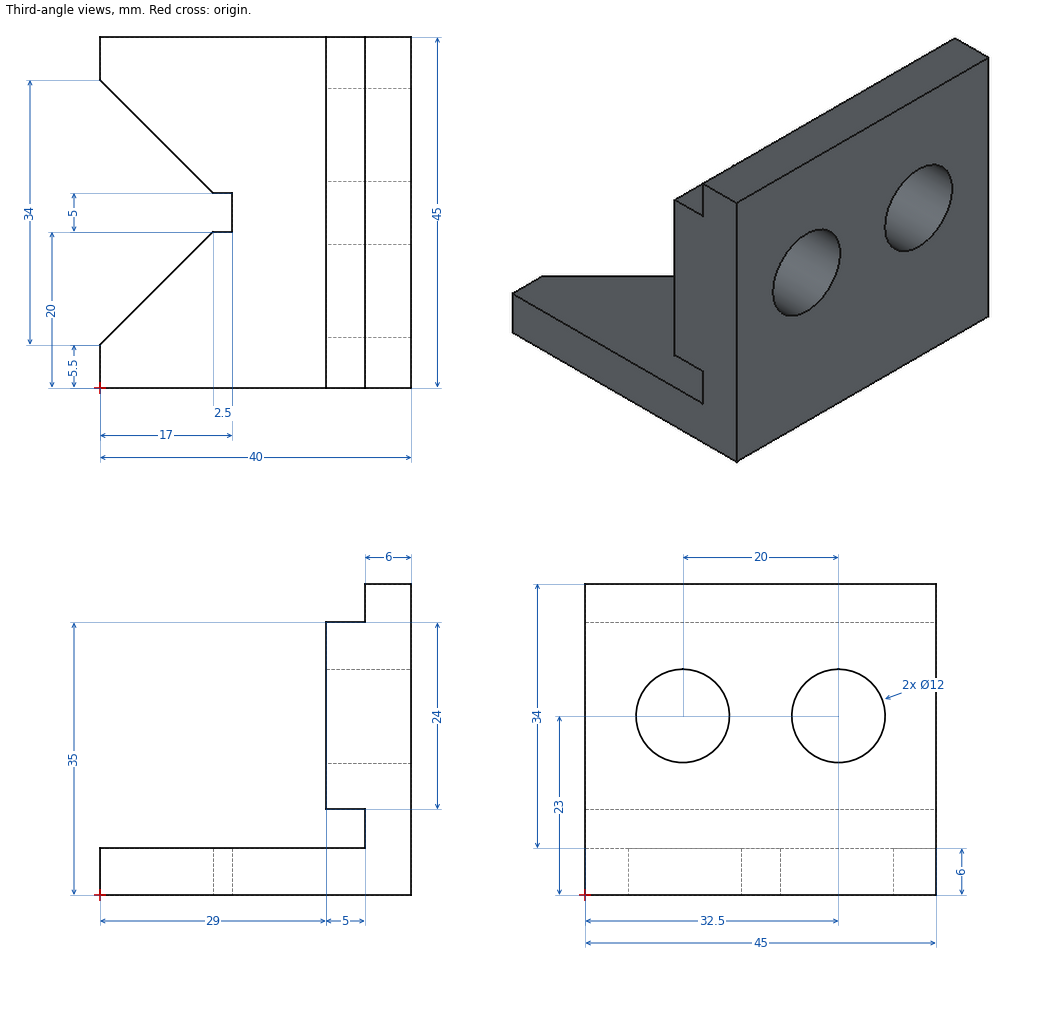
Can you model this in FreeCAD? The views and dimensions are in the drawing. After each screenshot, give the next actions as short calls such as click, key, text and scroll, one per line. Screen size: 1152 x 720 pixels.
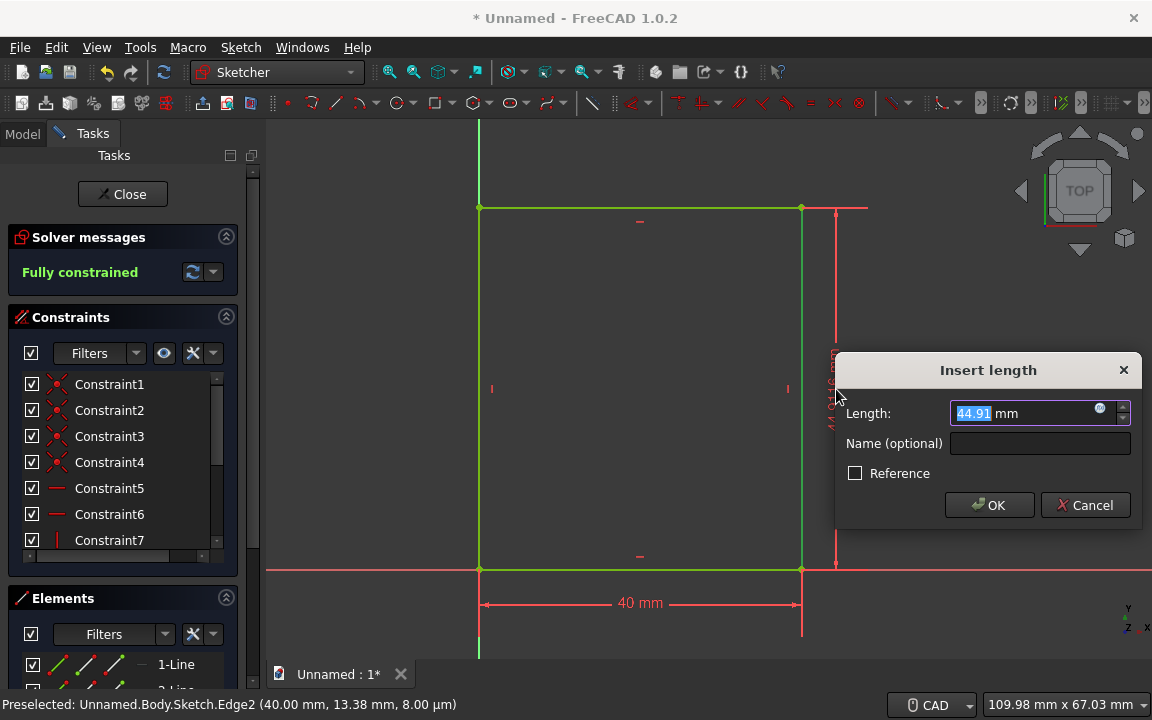
text(45)
key(Return)
key(Escape)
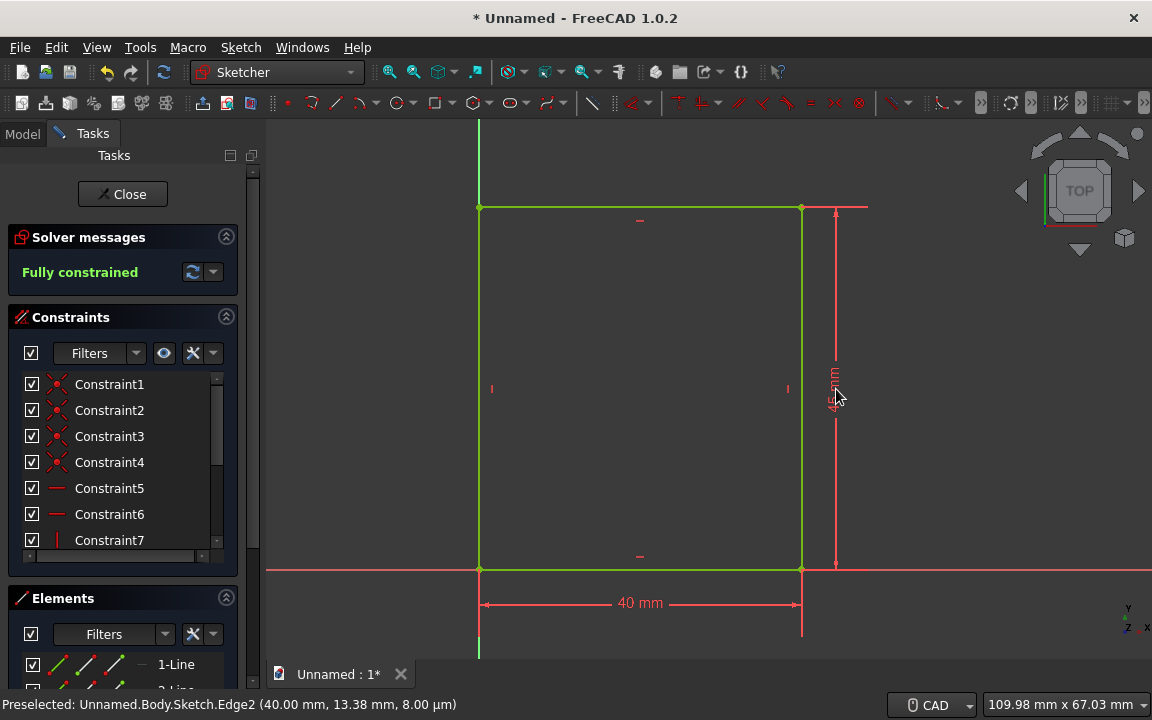
click(123, 194)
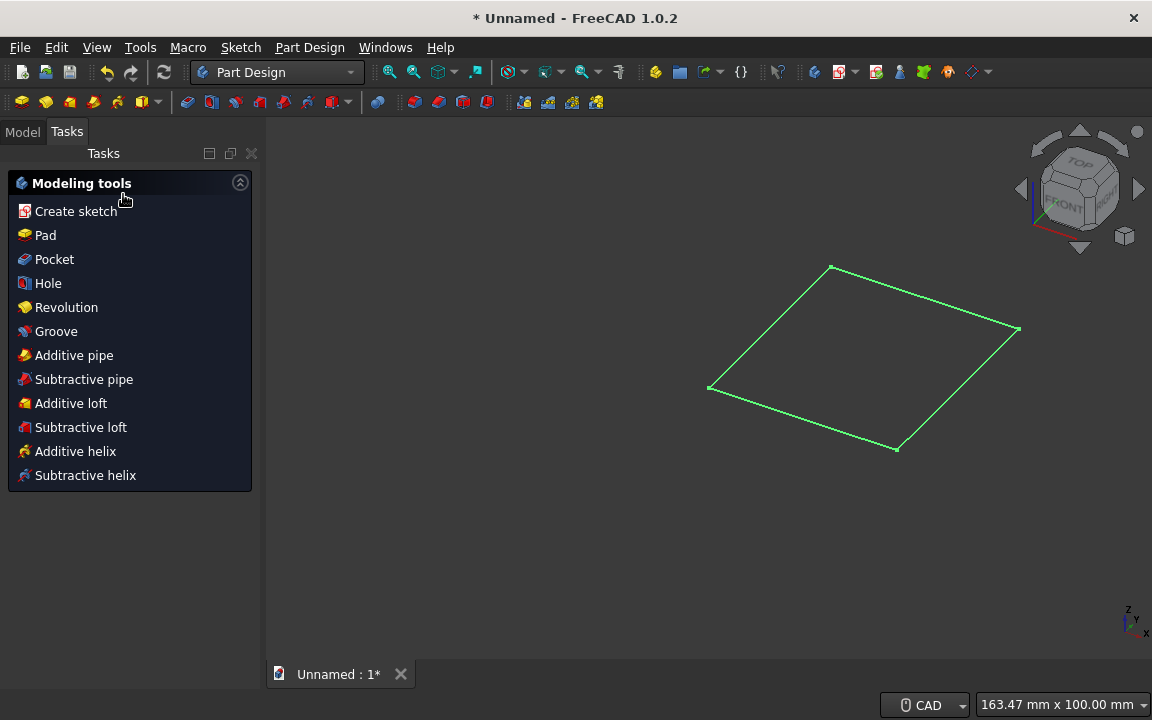
click(22, 102)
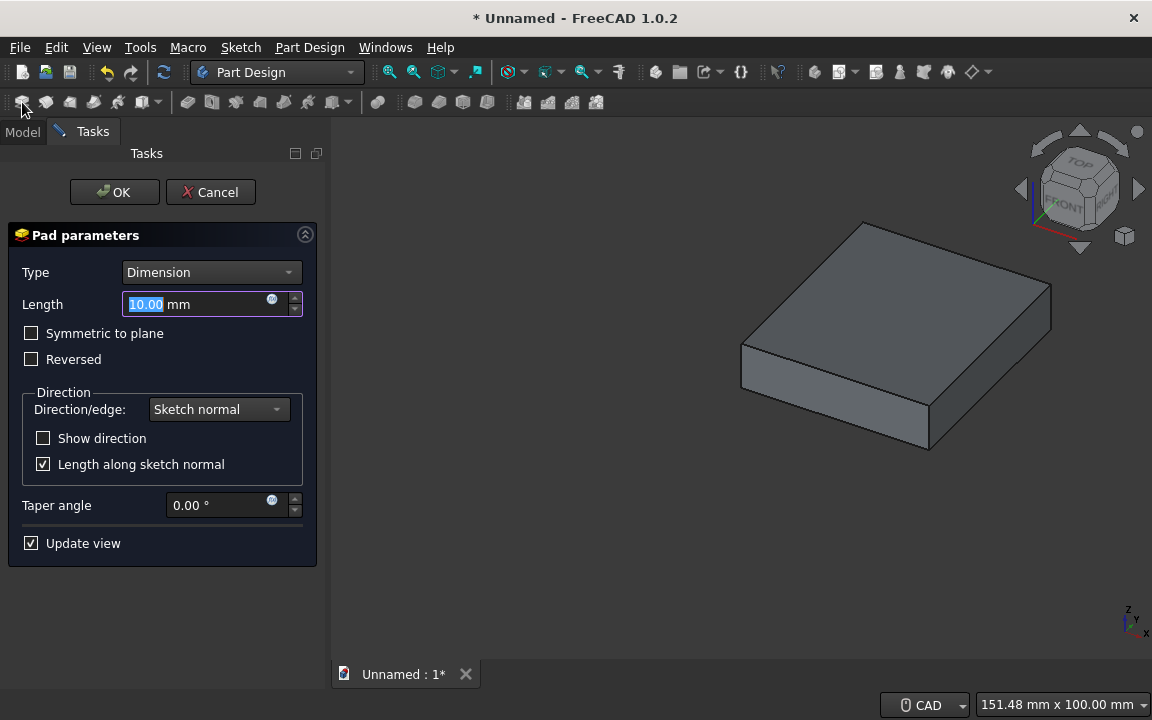
text(6)
key(Tab)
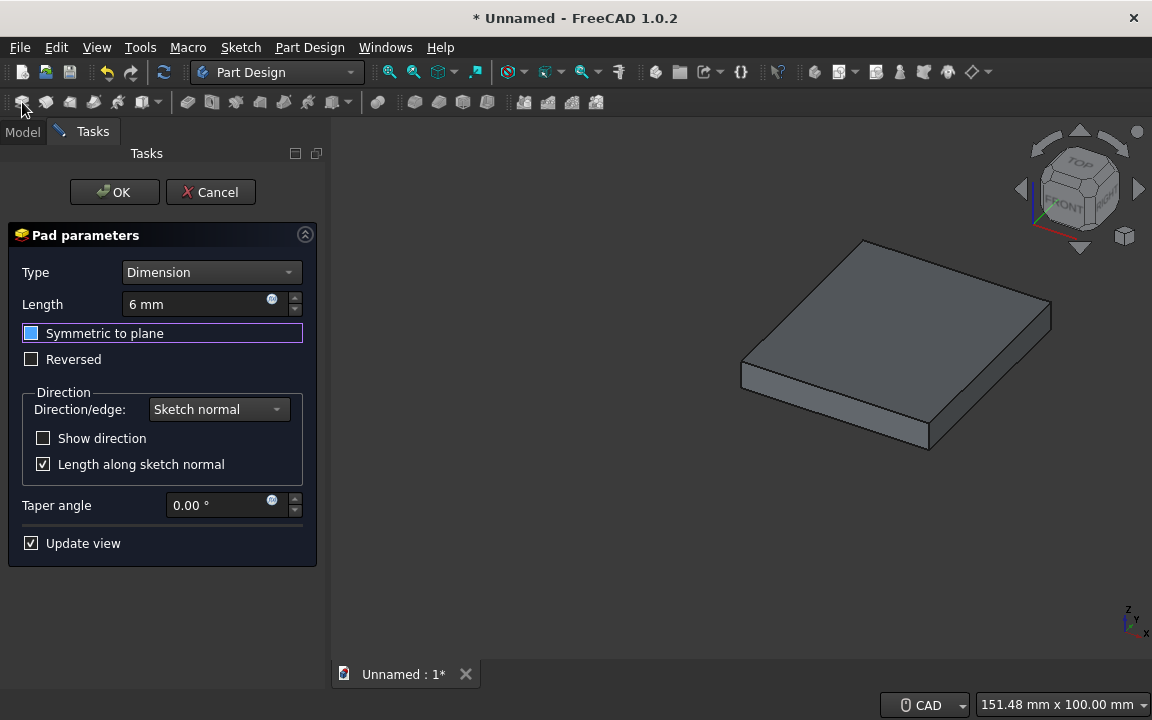
click(115, 192)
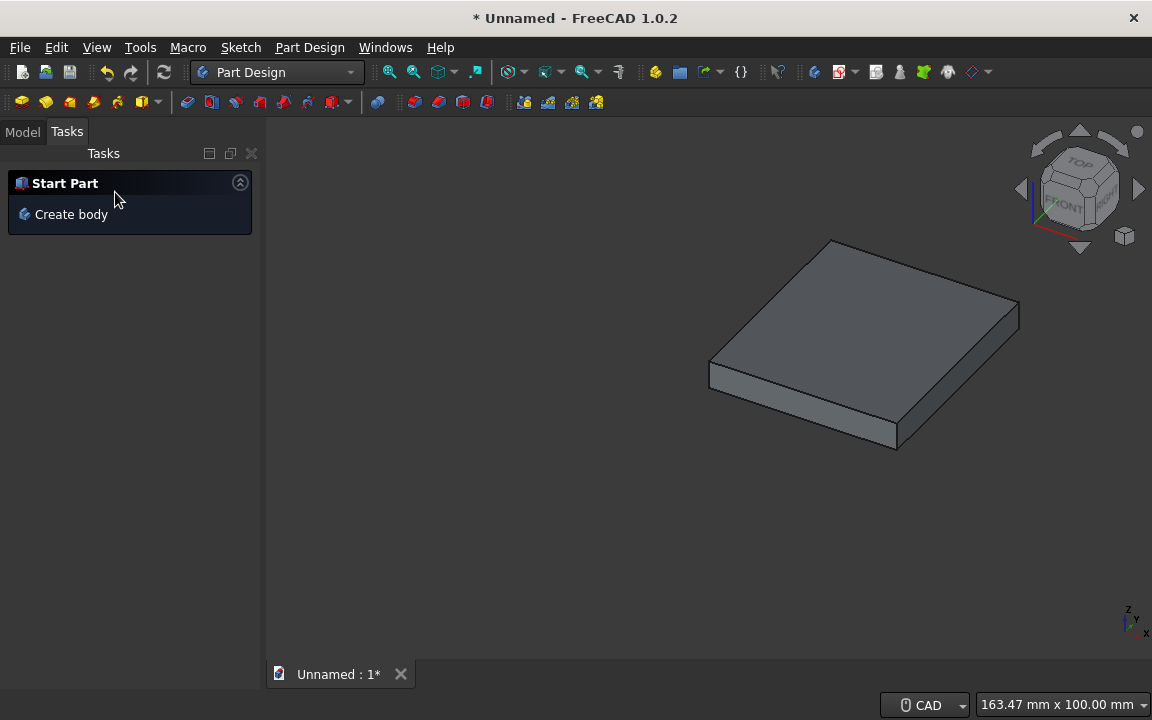
click(390, 72)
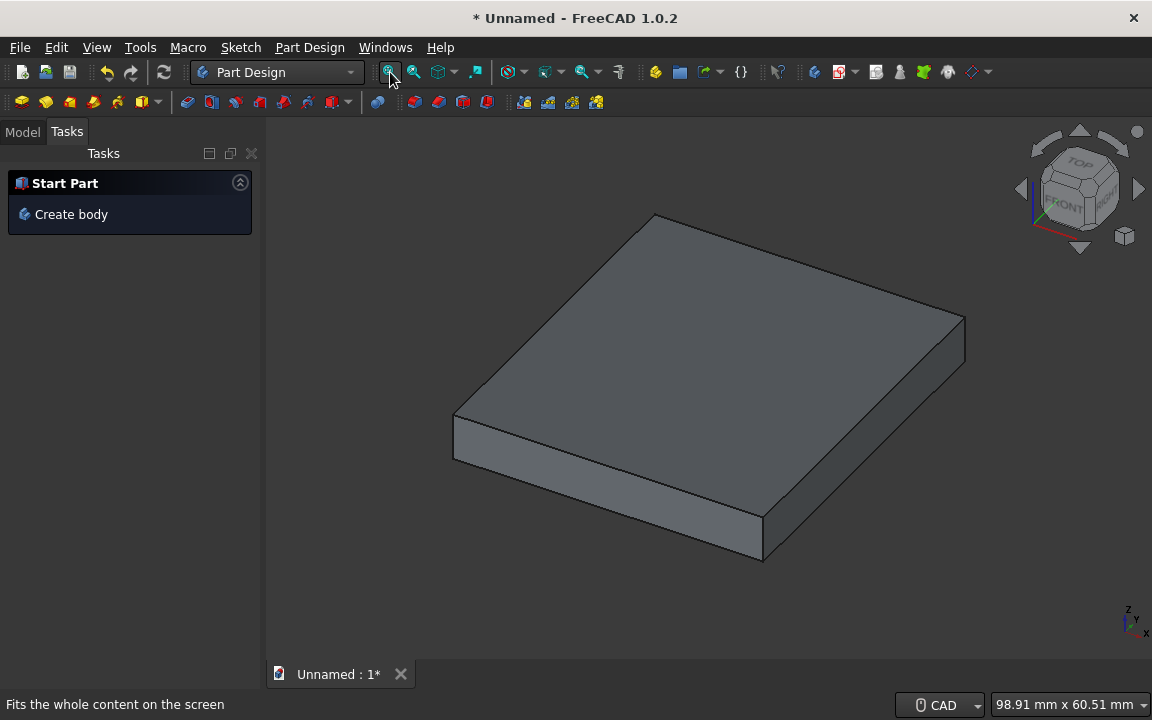
click(951, 353)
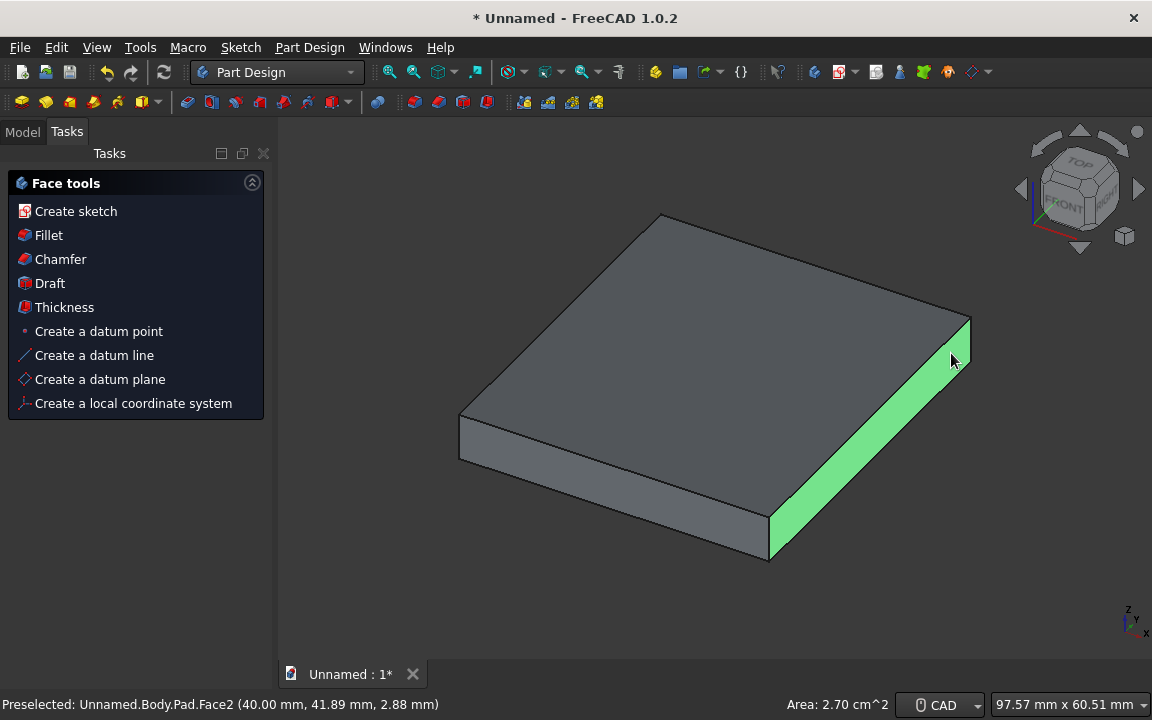
click(840, 72)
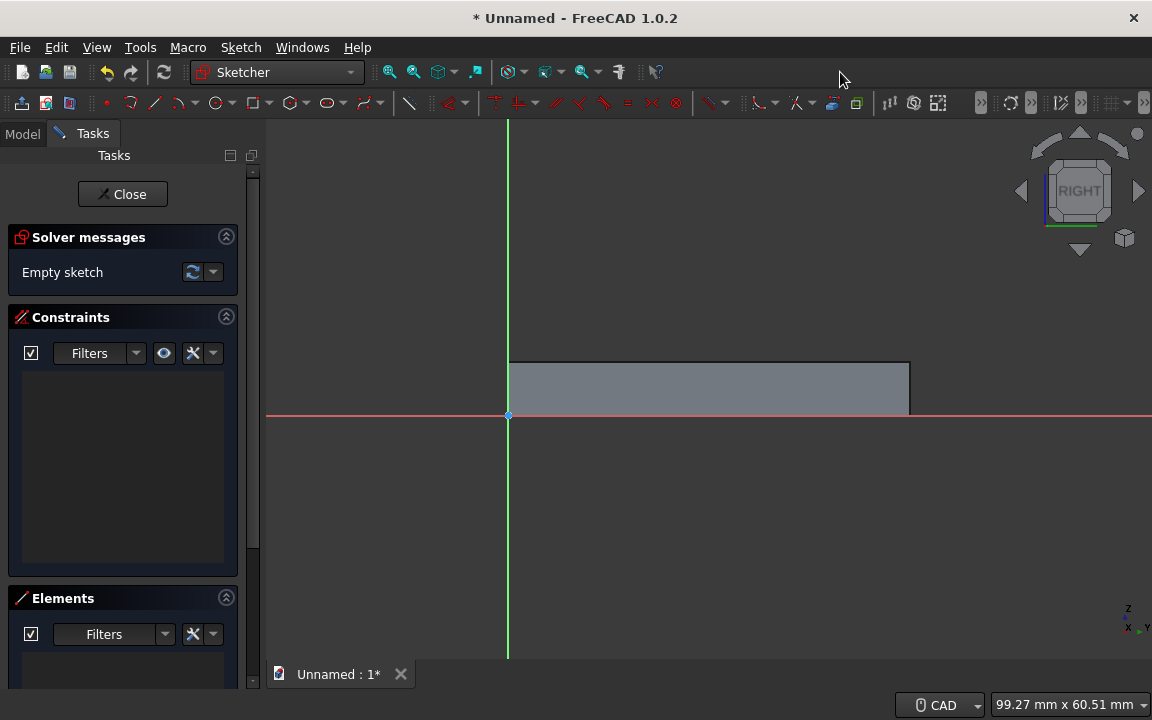
scroll(501, 631, down, 2)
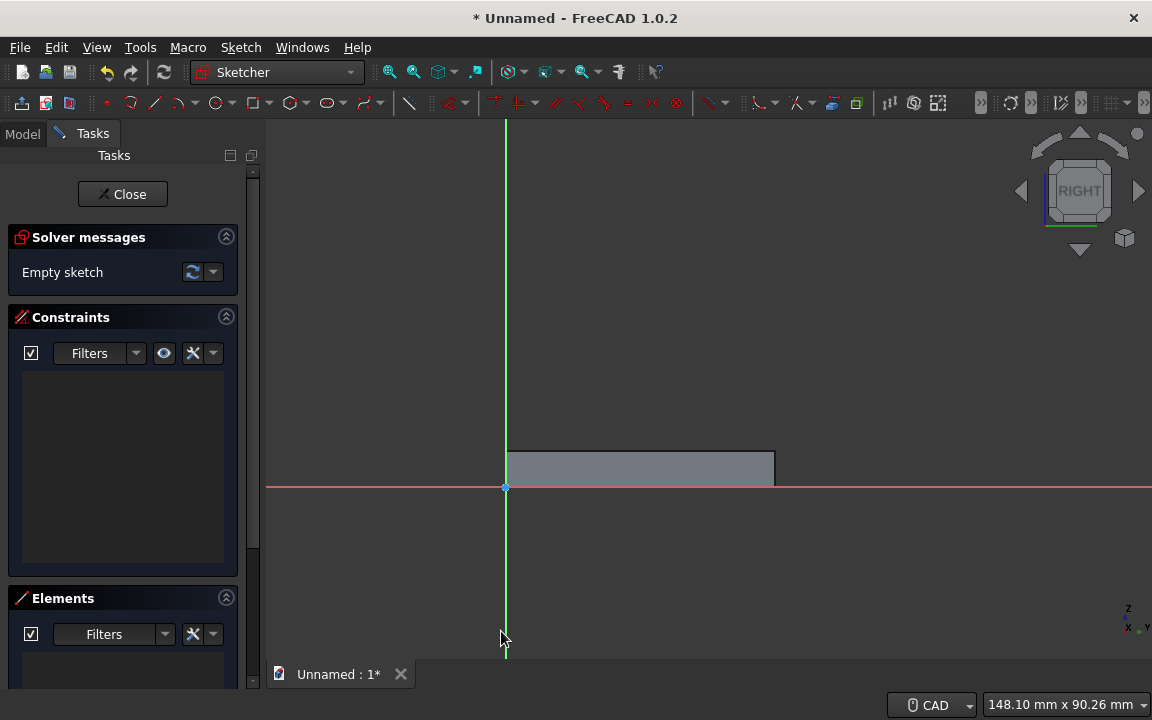
scroll(641, 323, up, 2)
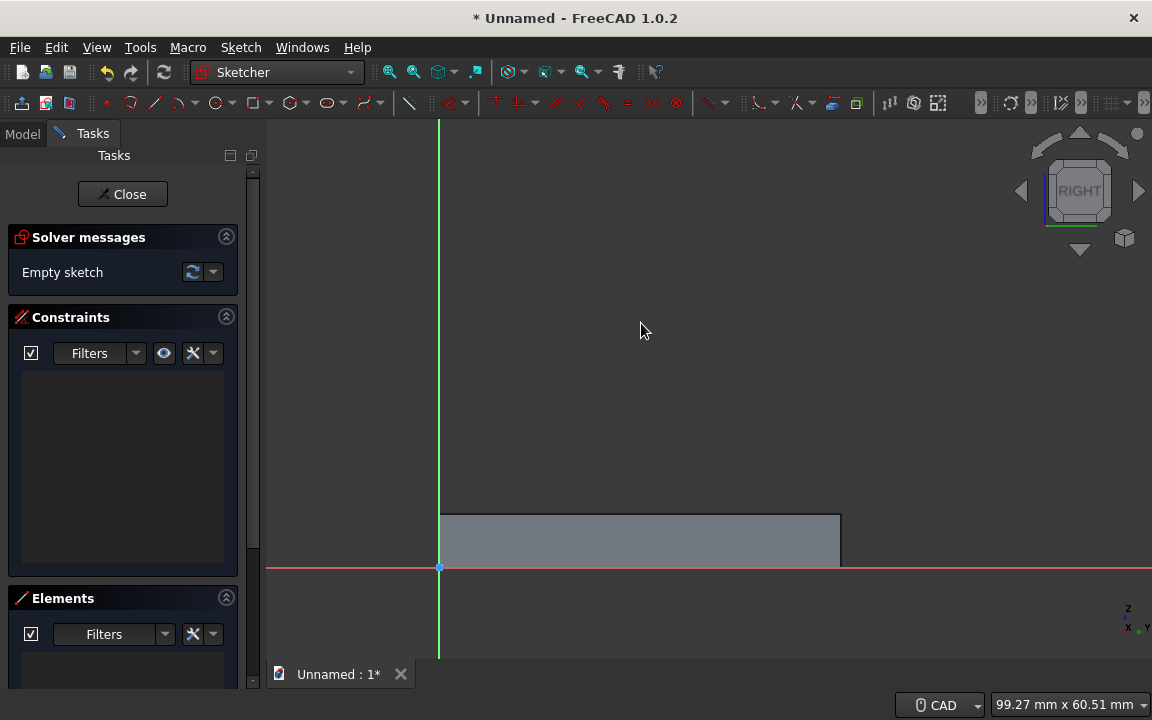
click(254, 104)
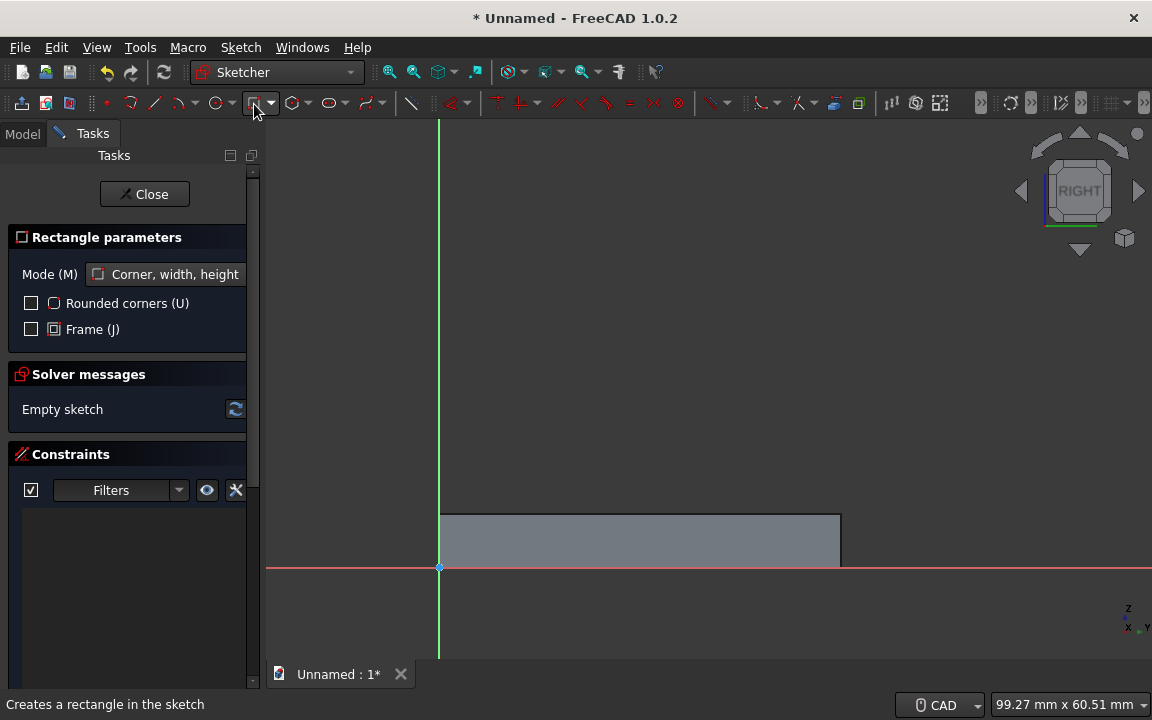
click(439, 211)
click(841, 514)
key(Escape)